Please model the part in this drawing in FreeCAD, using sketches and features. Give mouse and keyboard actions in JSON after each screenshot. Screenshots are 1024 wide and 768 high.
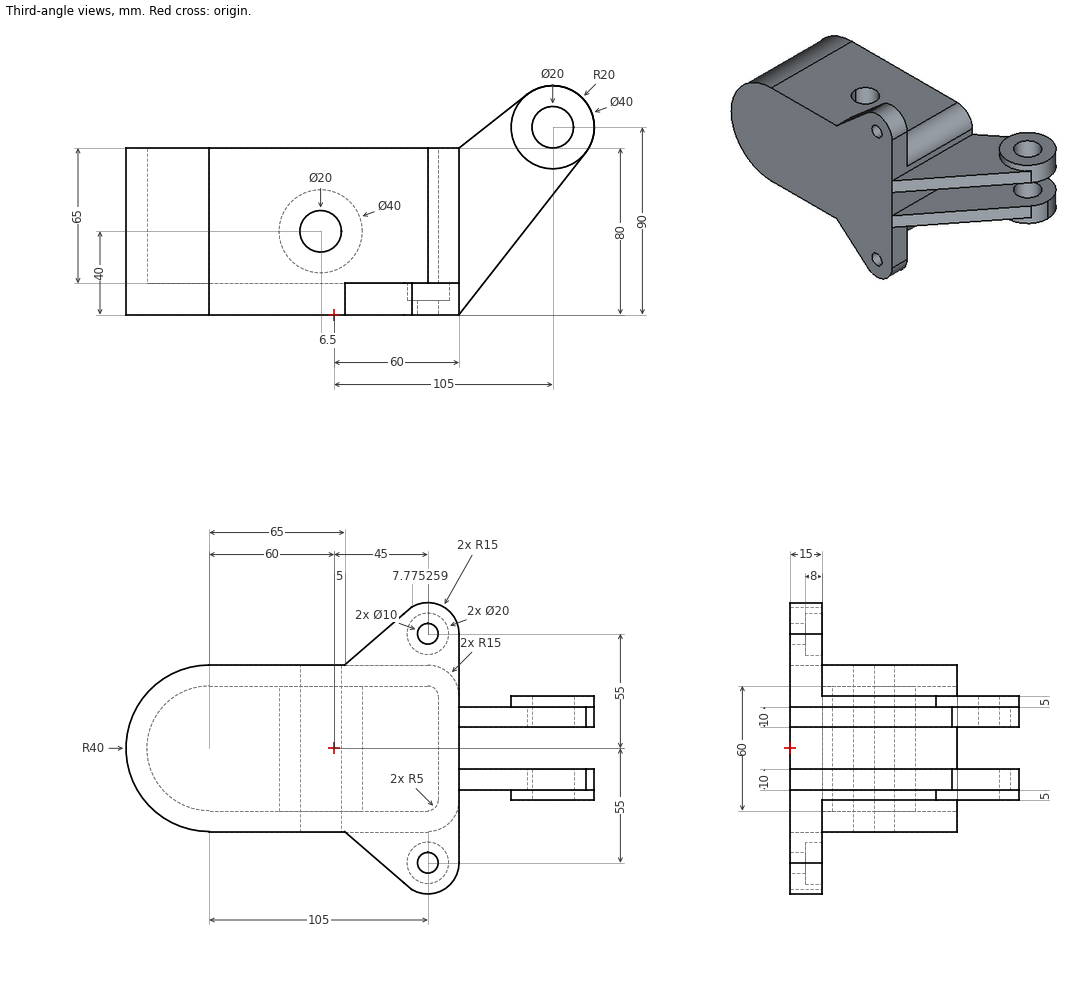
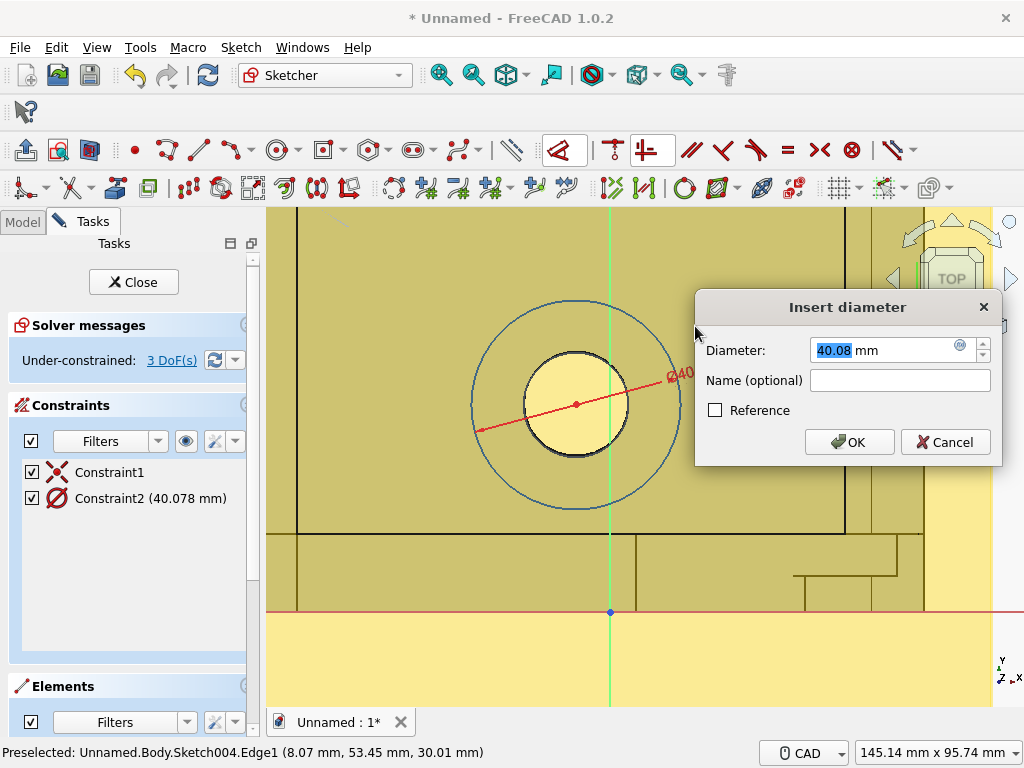
{"action": "type", "text": "40"}
{"action": "key", "text": "Return"}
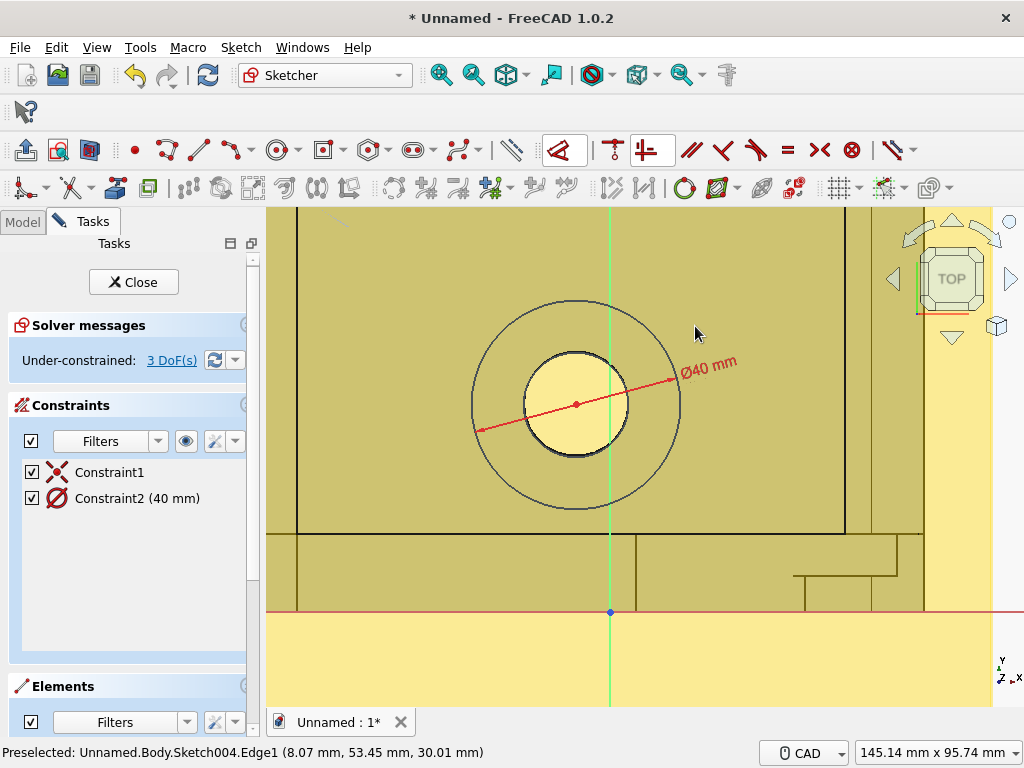
{"action": "left_click", "coordinate": [613, 368]}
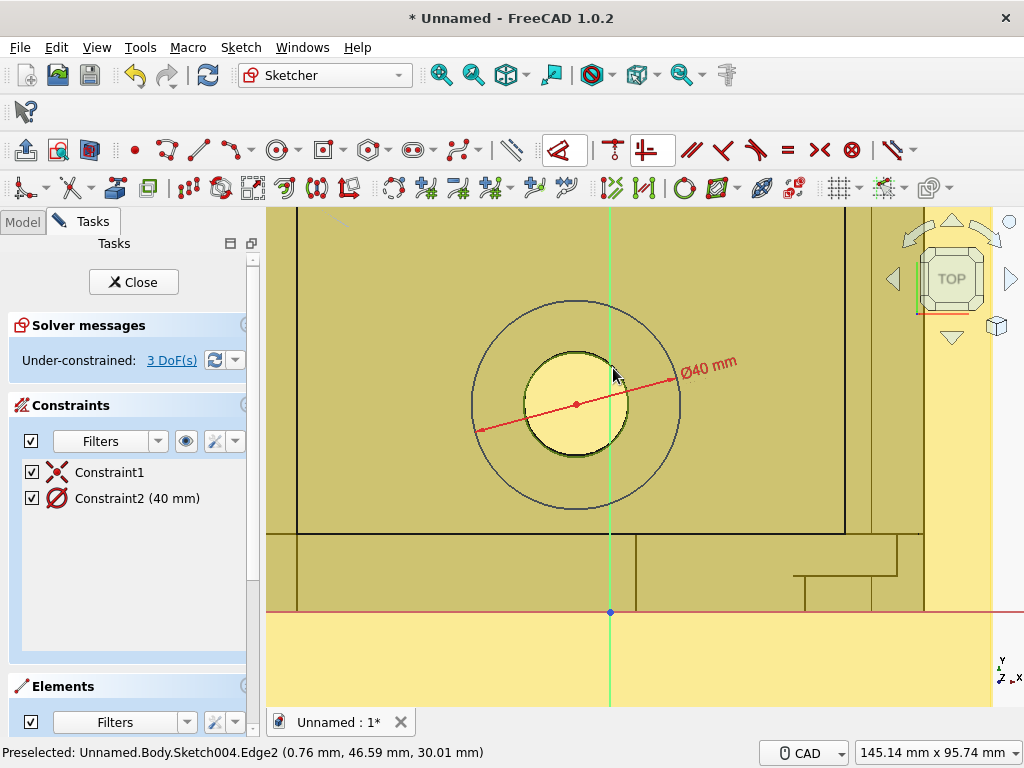
{"action": "left_click", "coordinate": [582, 150]}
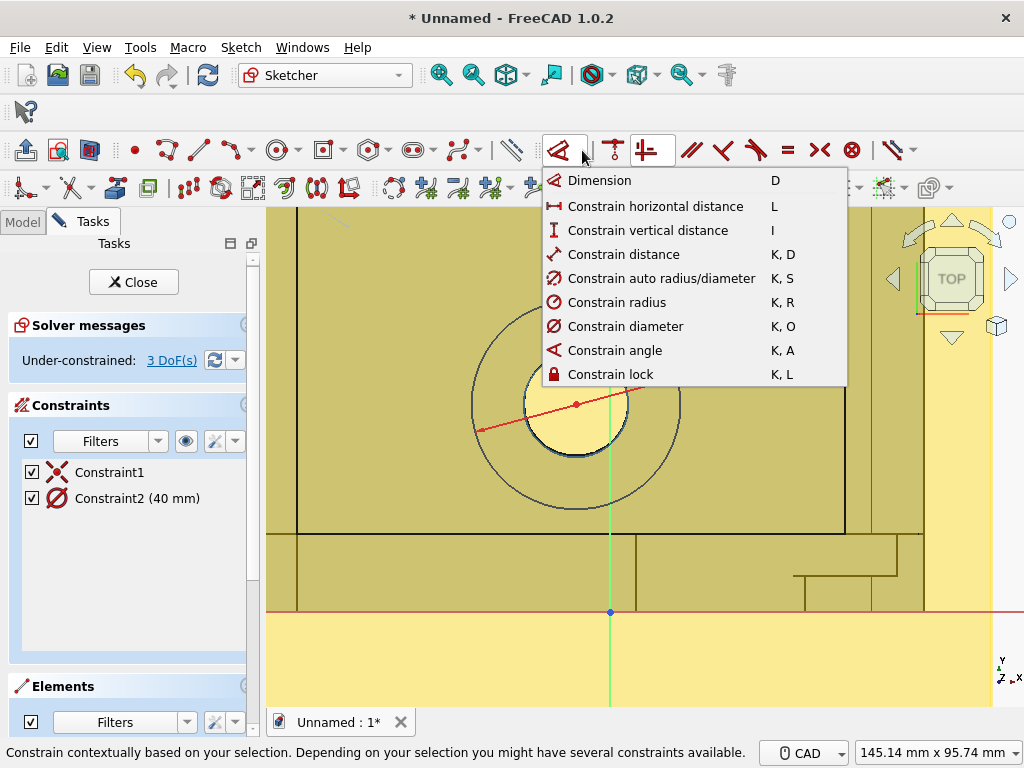
{"action": "left_click", "coordinate": [695, 326]}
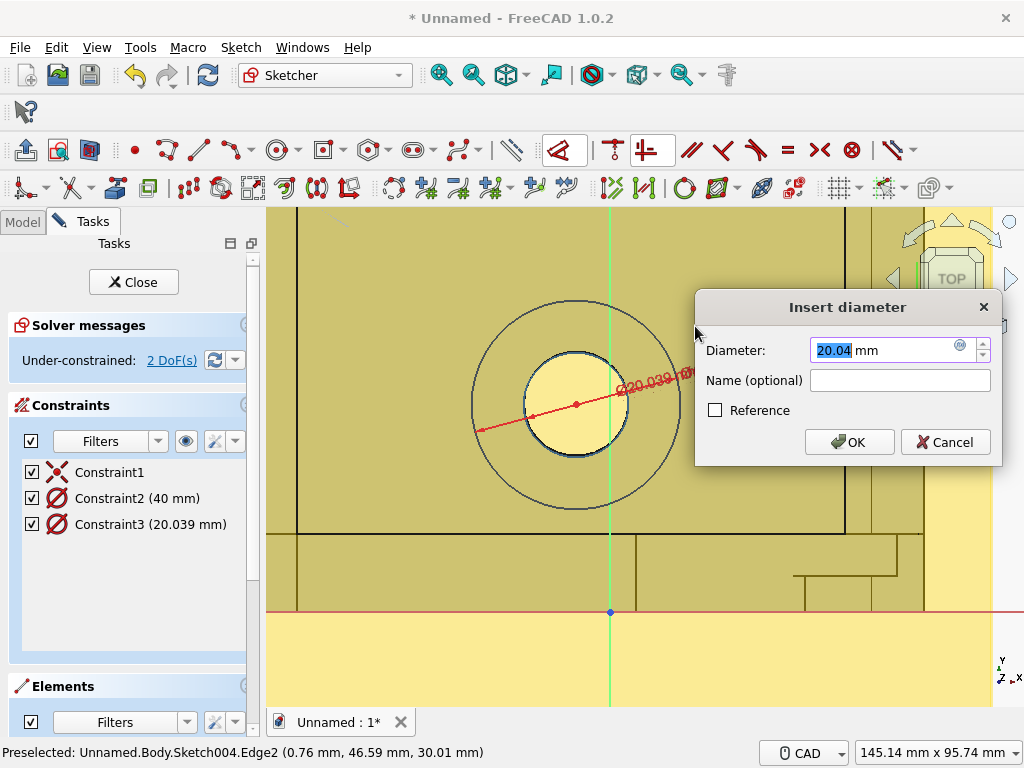
{"action": "type", "text": "20"}
{"action": "key", "text": "Return"}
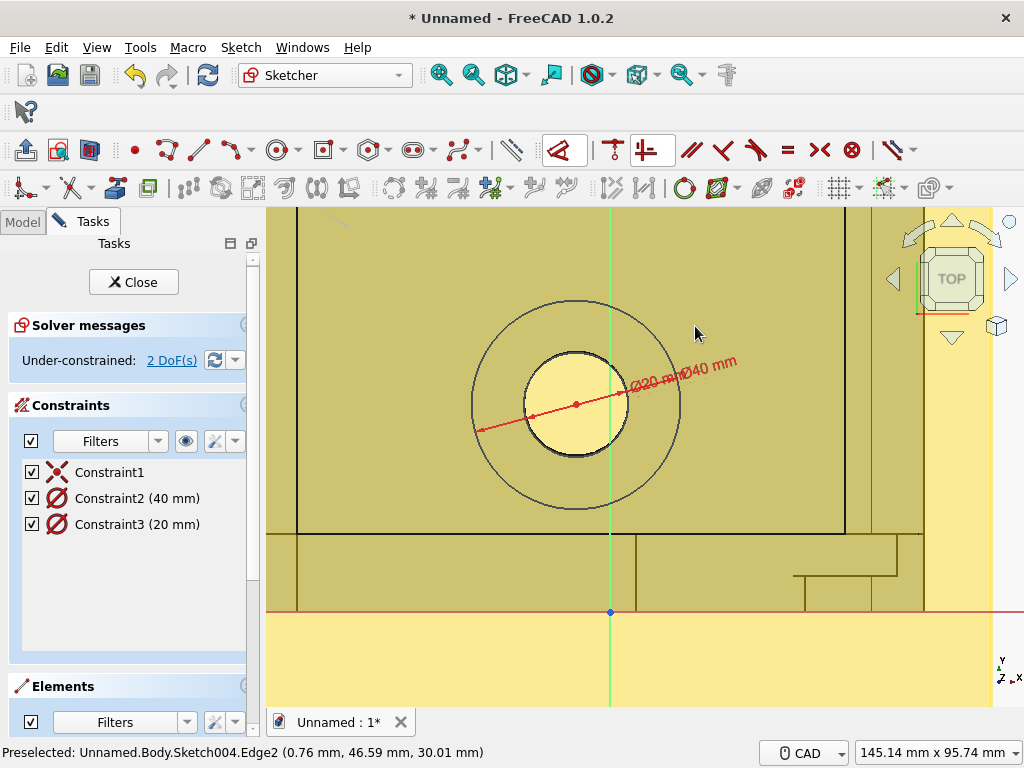
{"action": "left_click", "coordinate": [576, 405]}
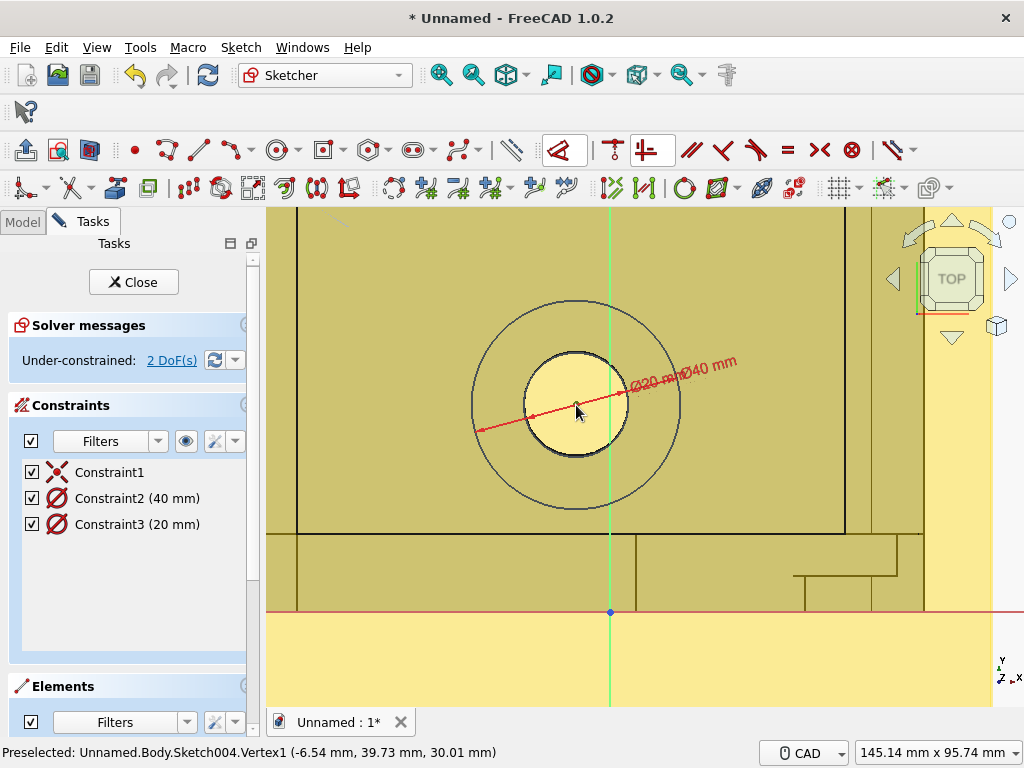
{"action": "left_click", "coordinate": [582, 150]}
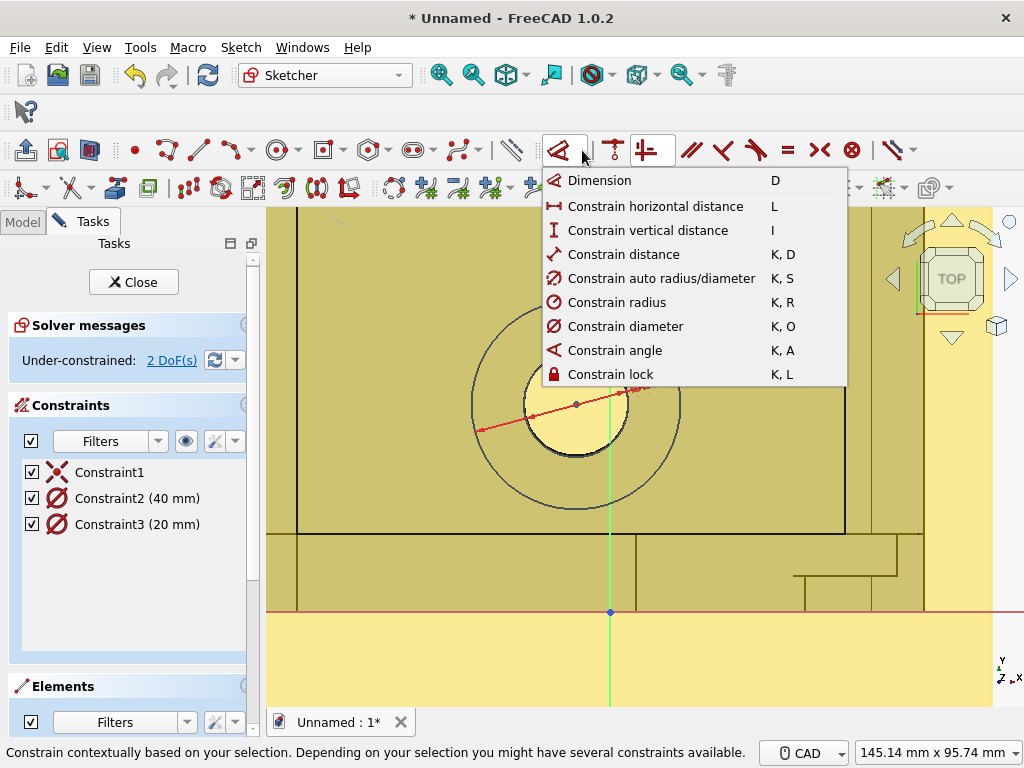
{"action": "left_click", "coordinate": [695, 230]}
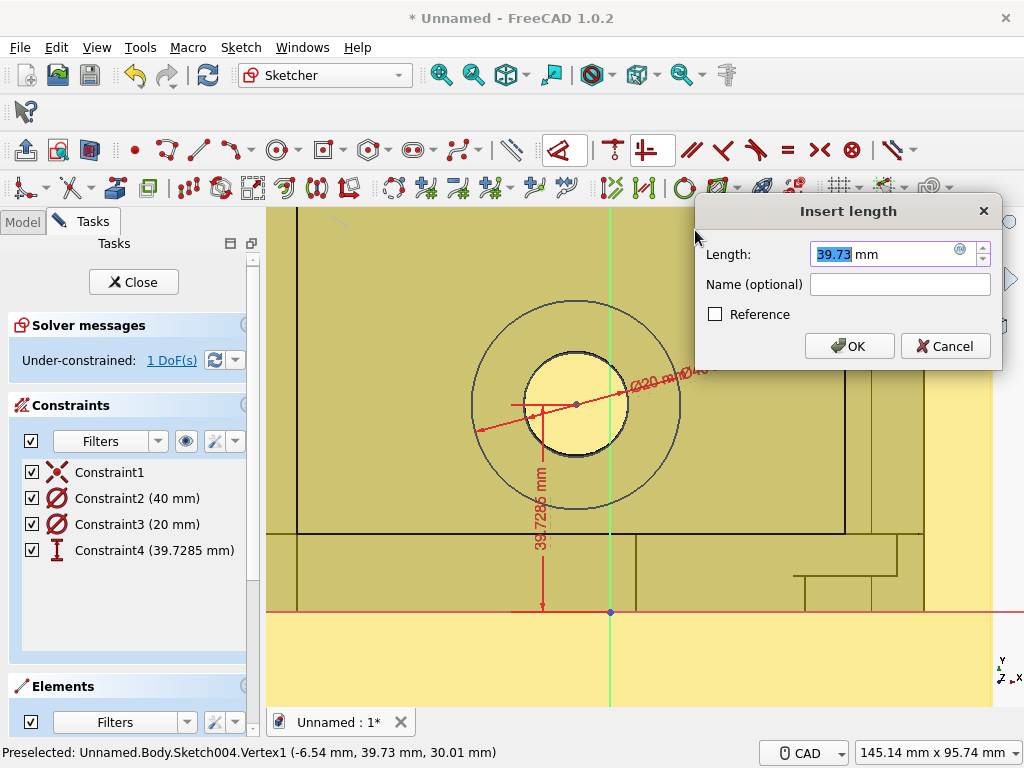
{"action": "type", "text": "40"}
{"action": "key", "text": "Return"}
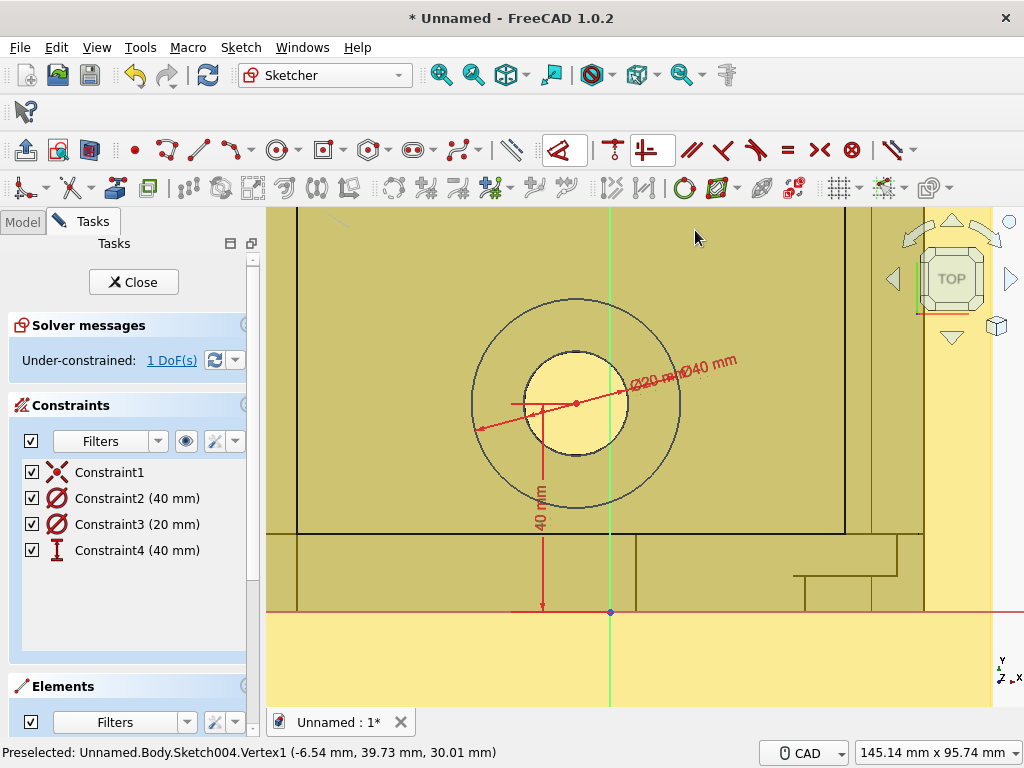
{"action": "left_click", "coordinate": [576, 404]}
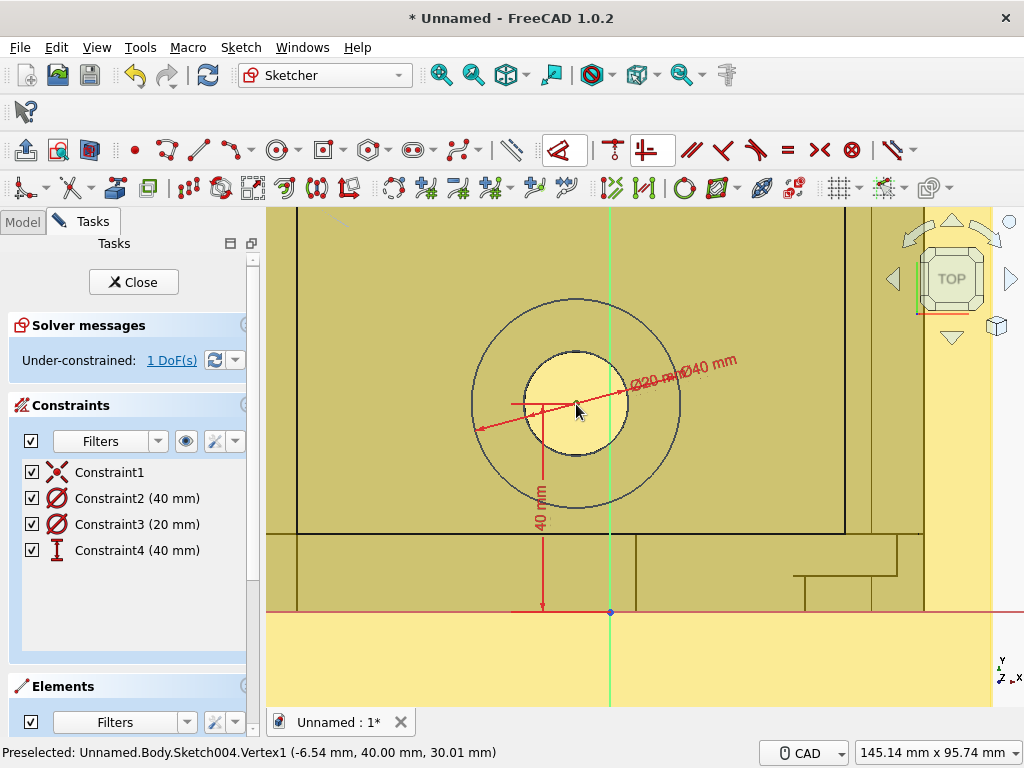
{"action": "key", "text": "l"}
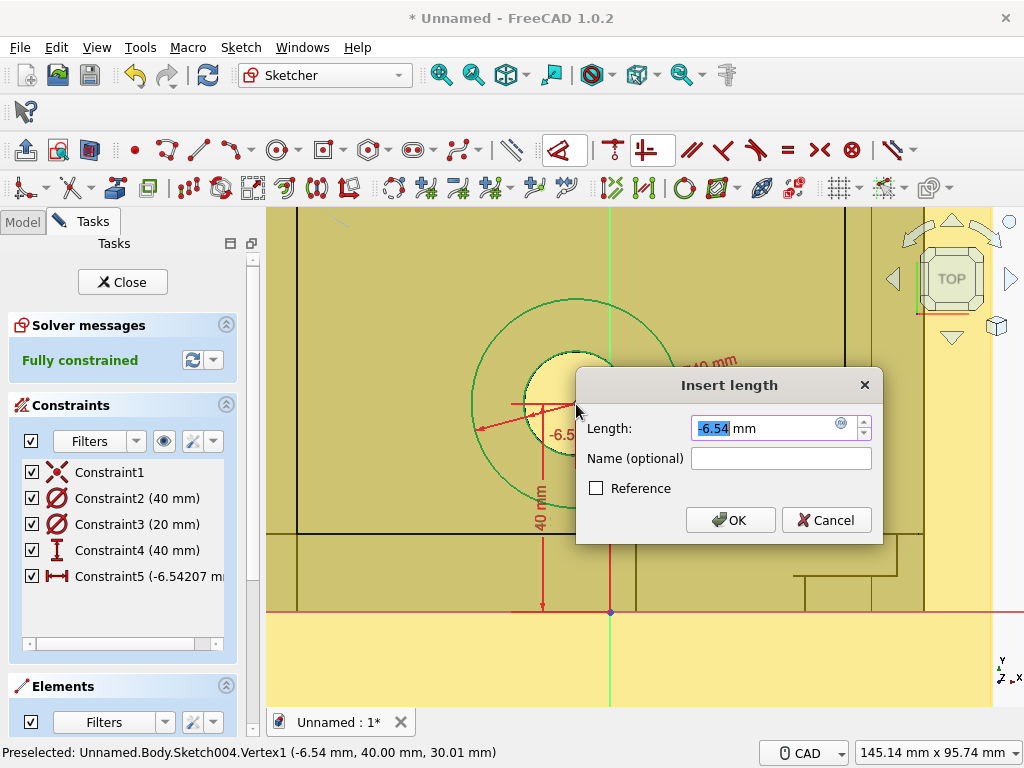
{"action": "type", "text": "-6.5"}
{"action": "key", "text": "Return"}